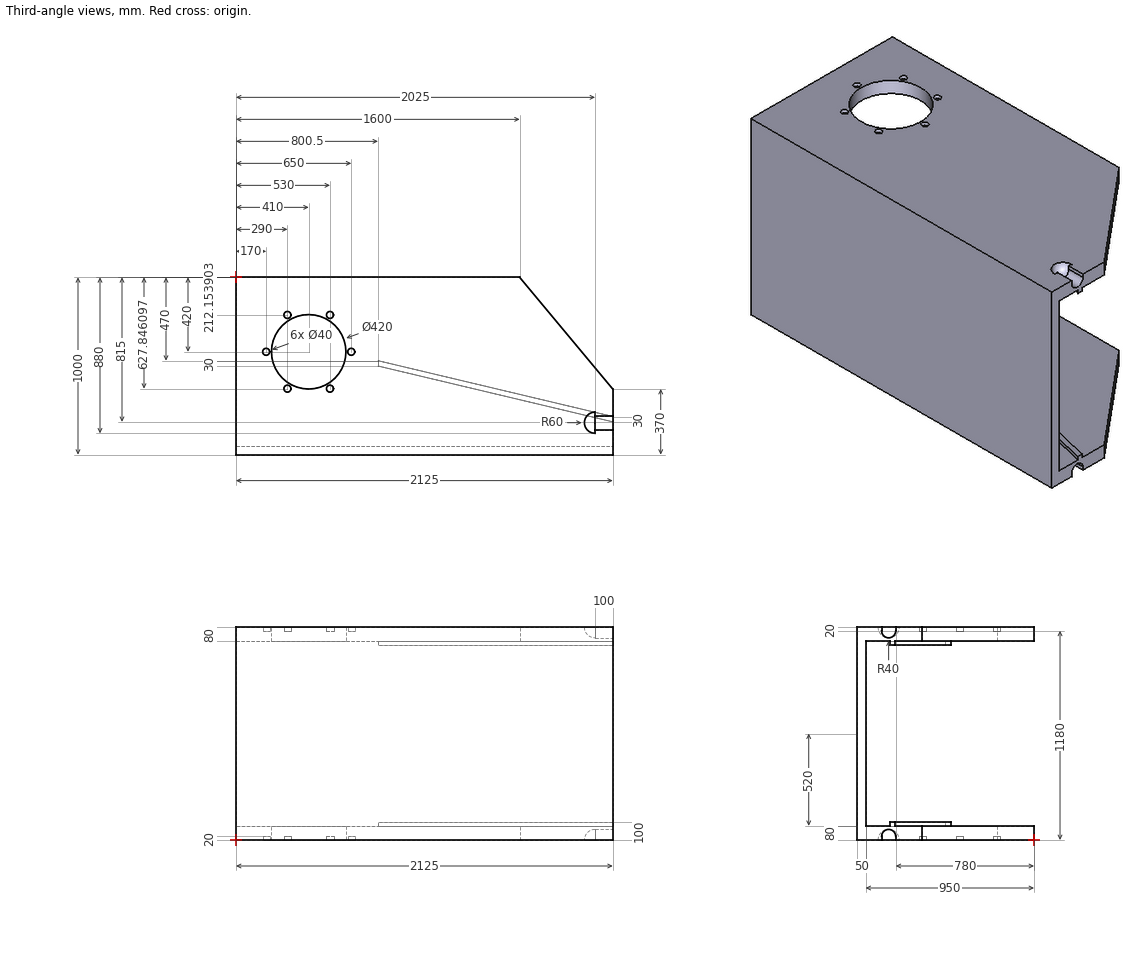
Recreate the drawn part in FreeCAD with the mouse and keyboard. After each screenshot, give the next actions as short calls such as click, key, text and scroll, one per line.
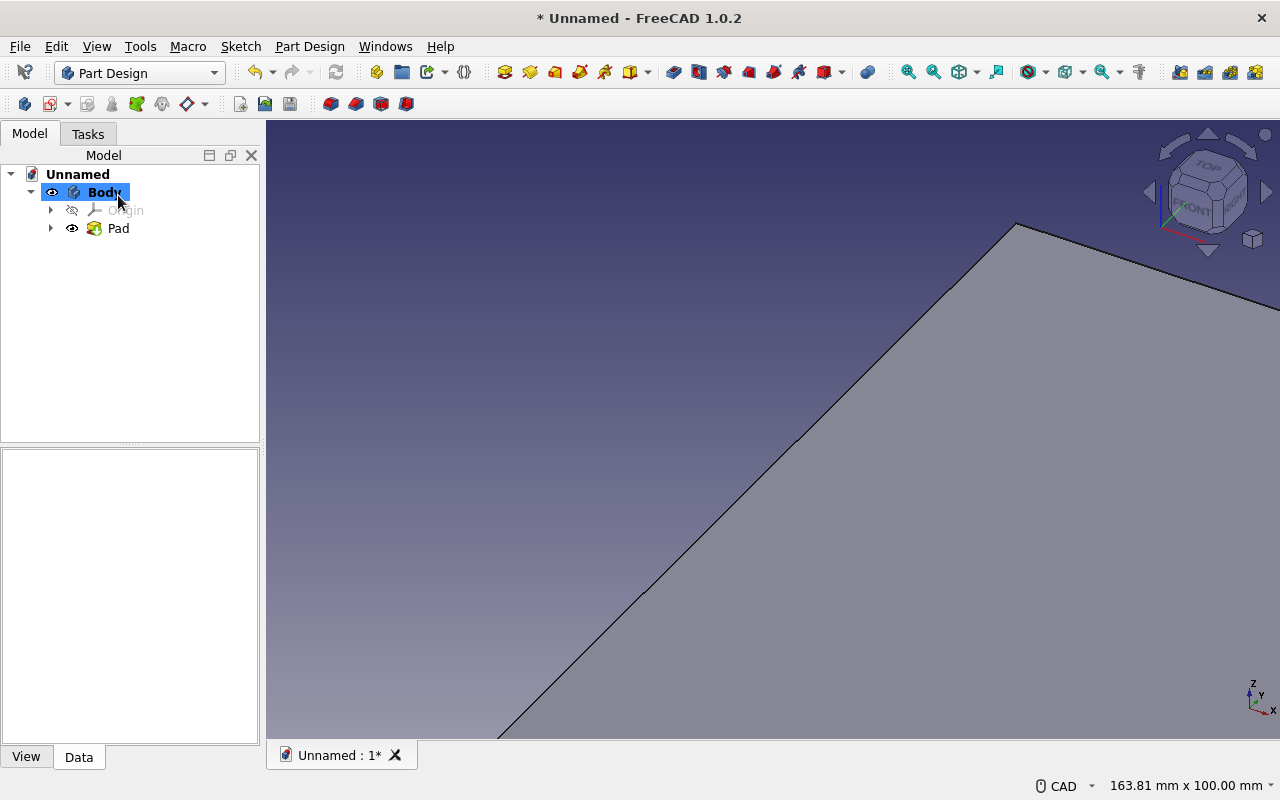
click(909, 72)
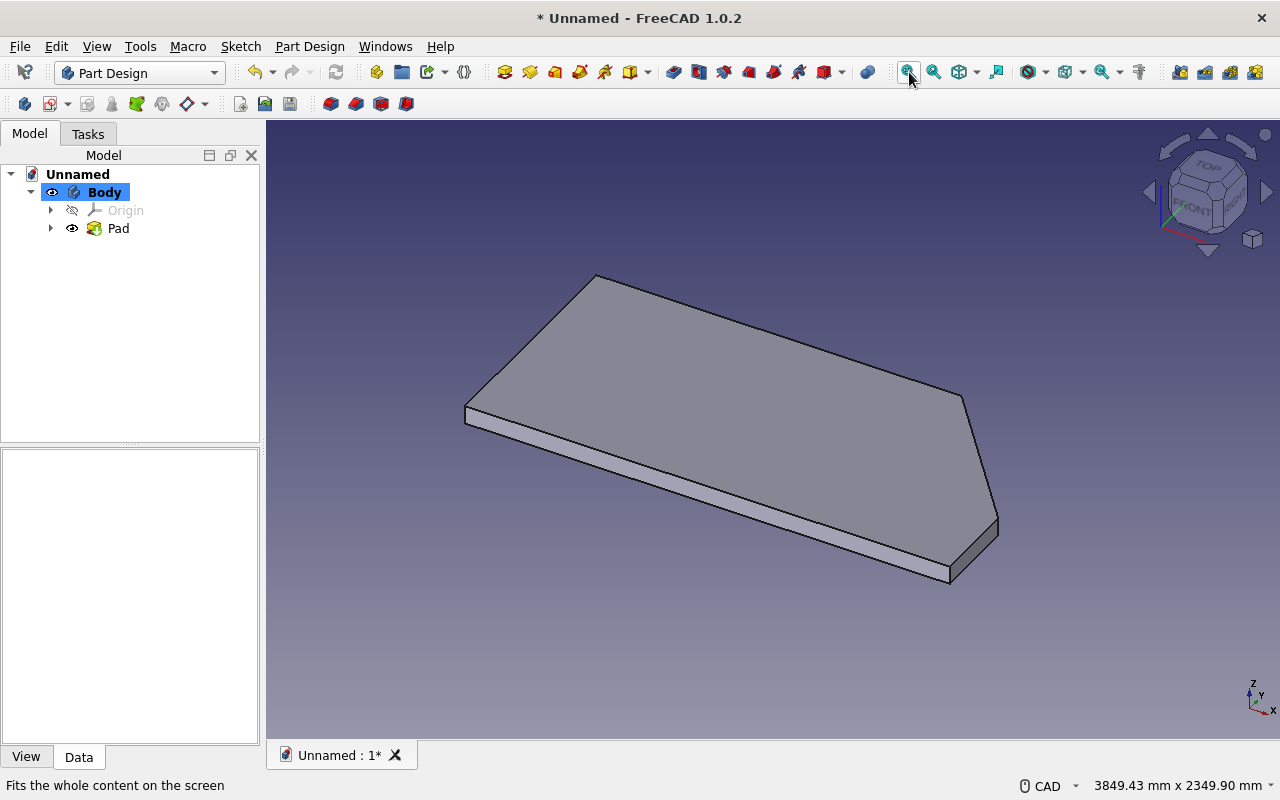
click(50, 104)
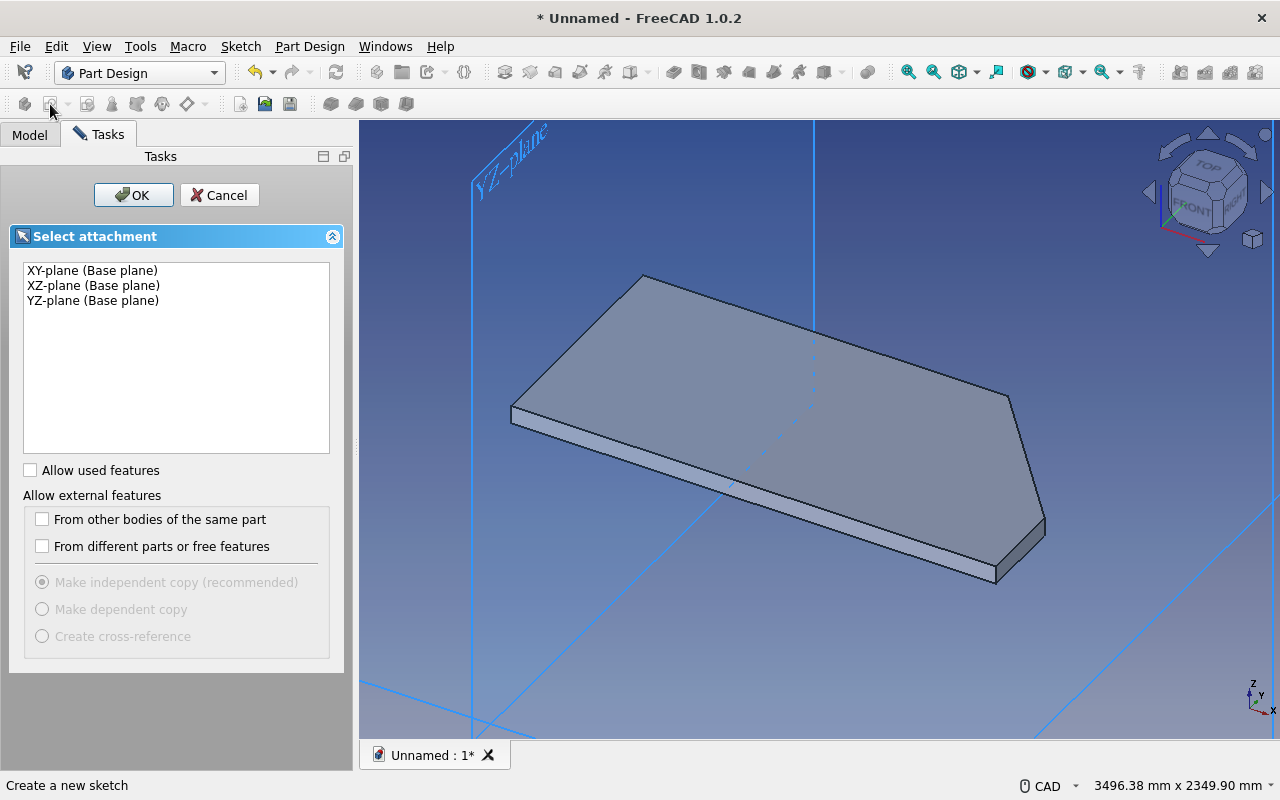
click(84, 300)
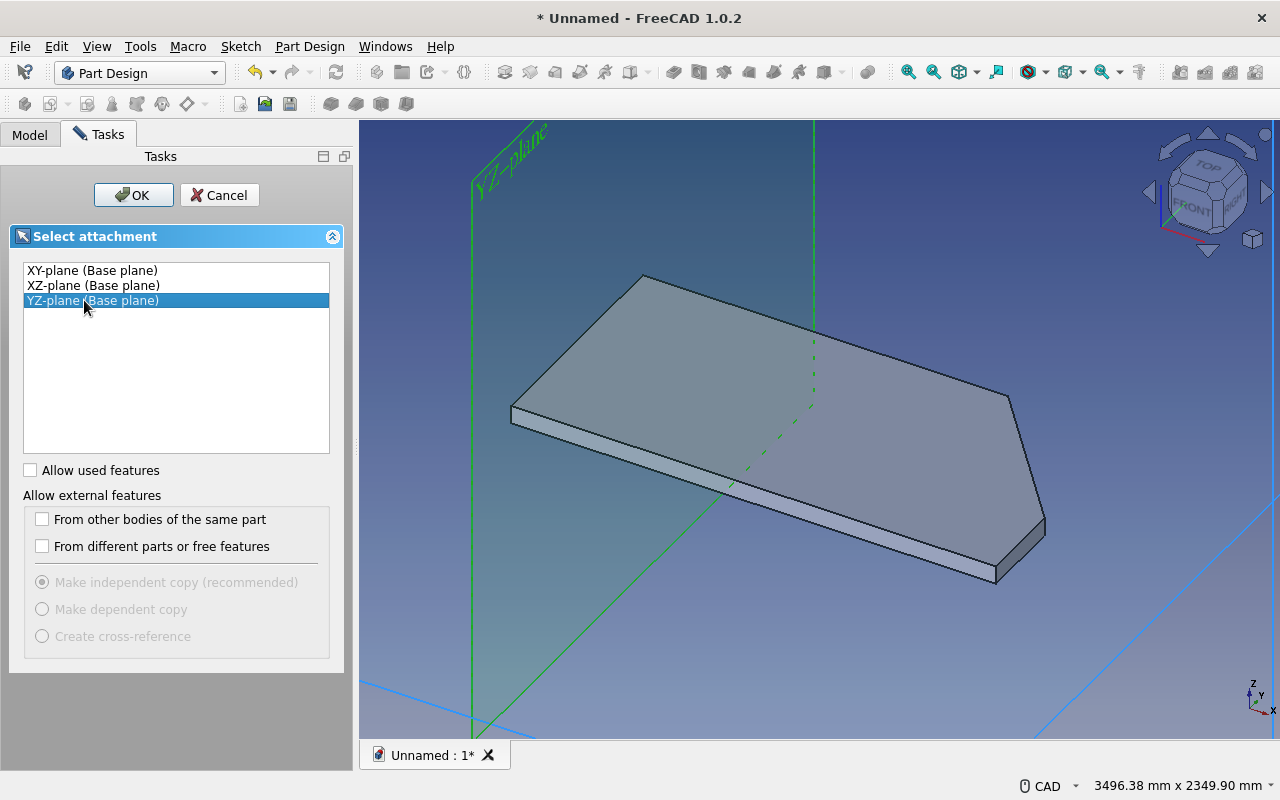
click(134, 195)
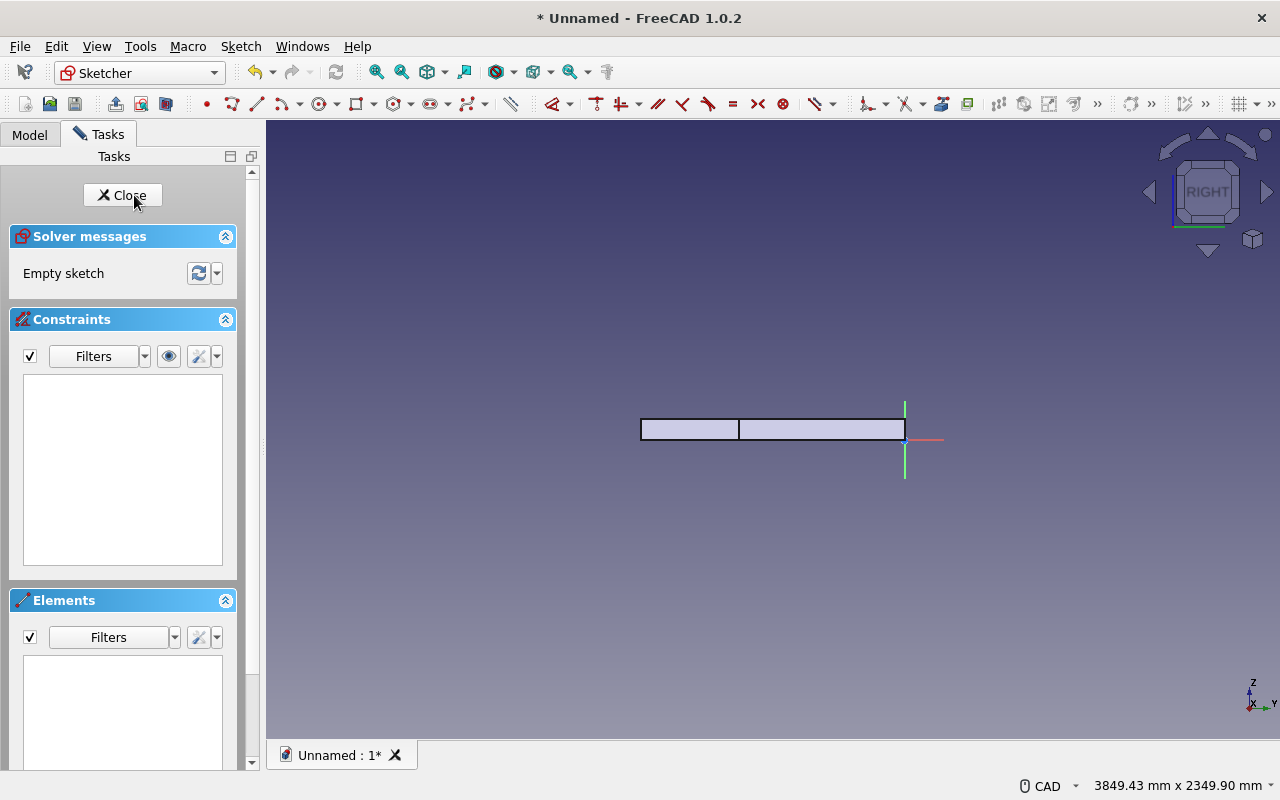
key(q)
key(s)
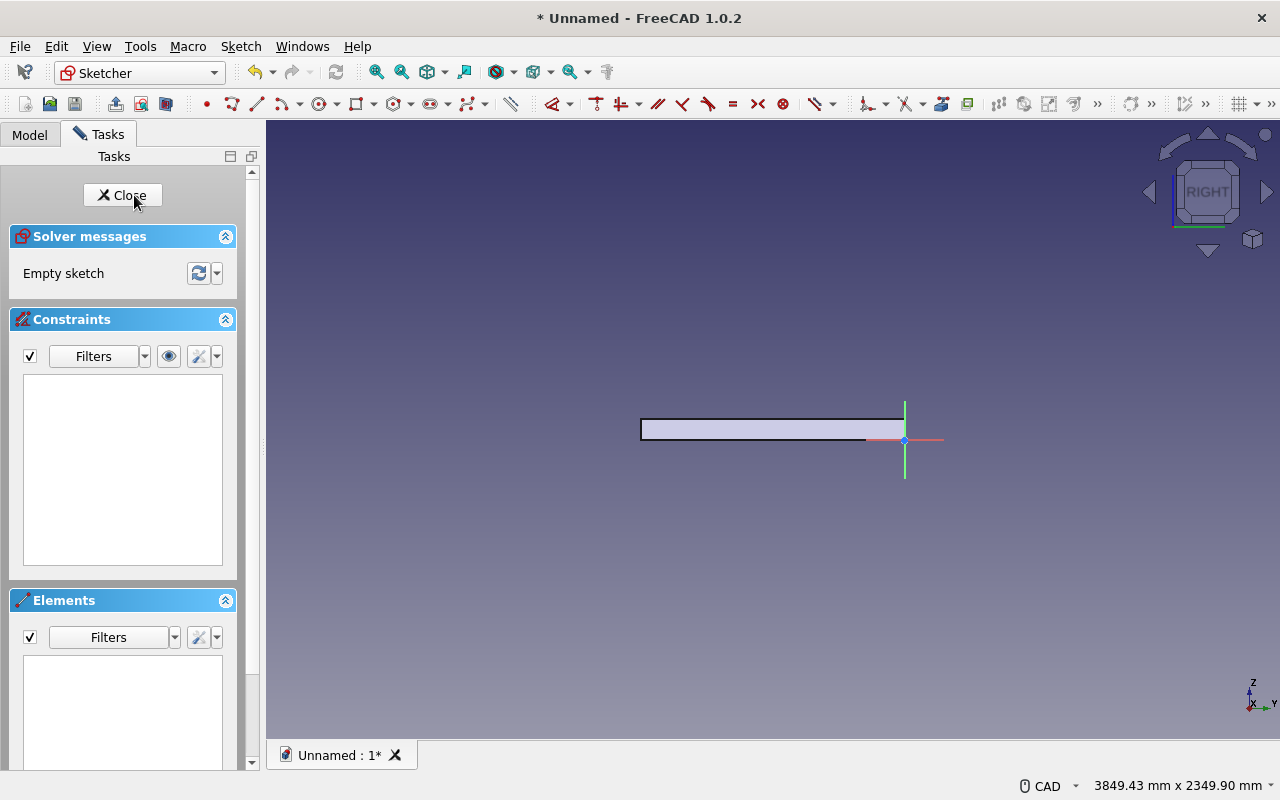
scroll(829, 305, up, 4)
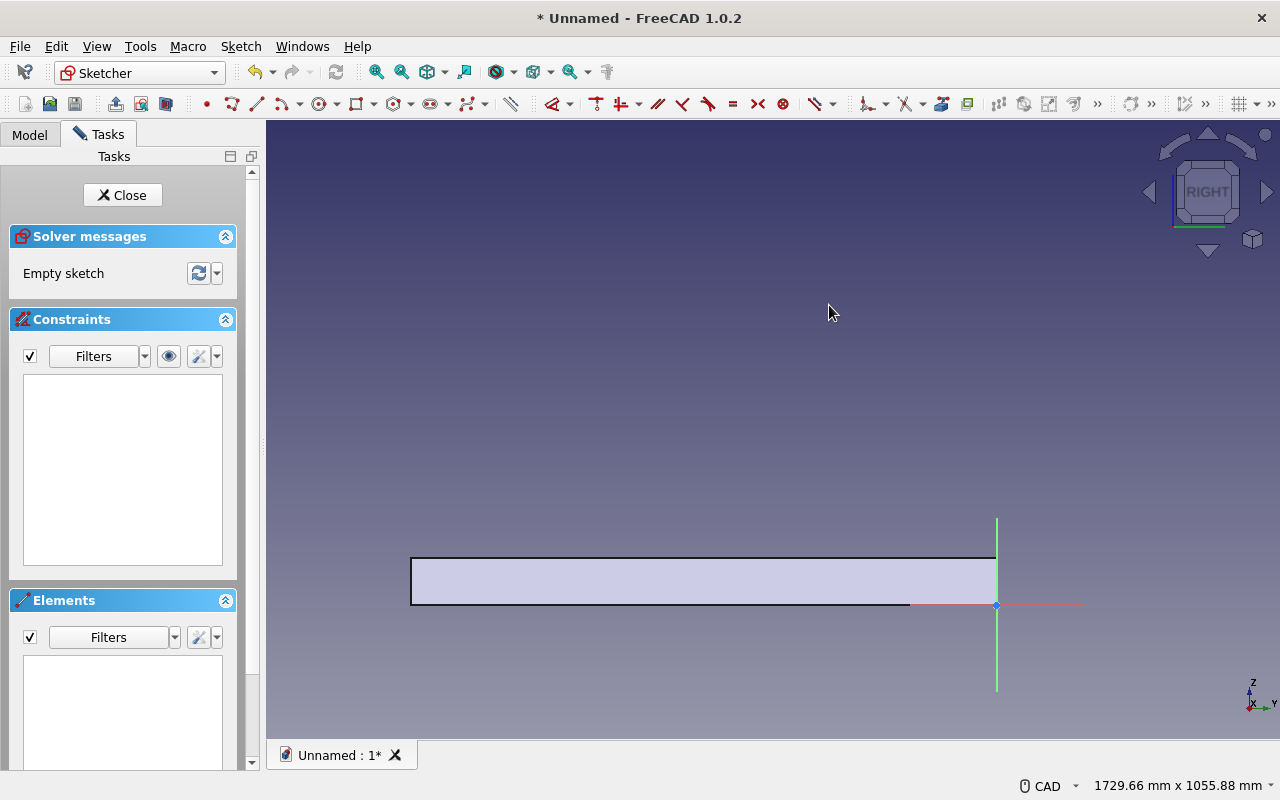
click(356, 104)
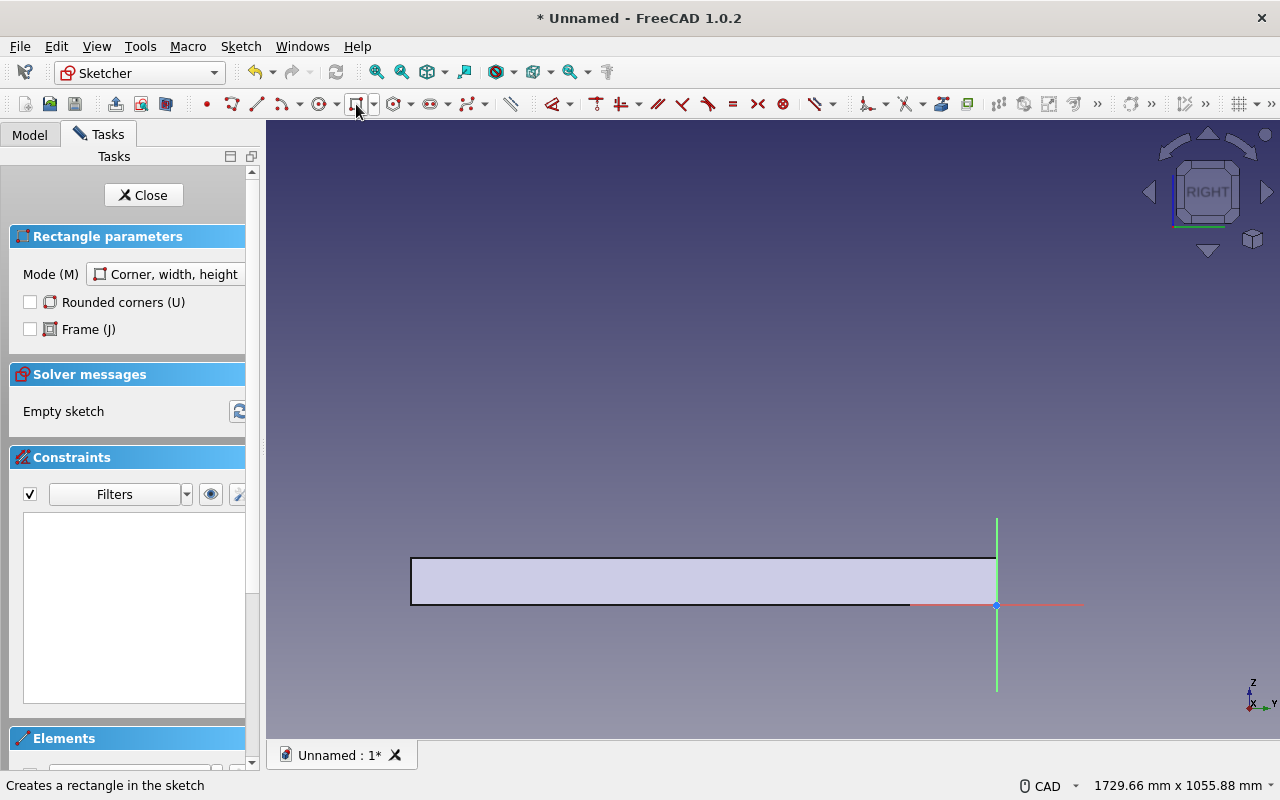
click(411, 253)
click(440, 558)
key(Escape)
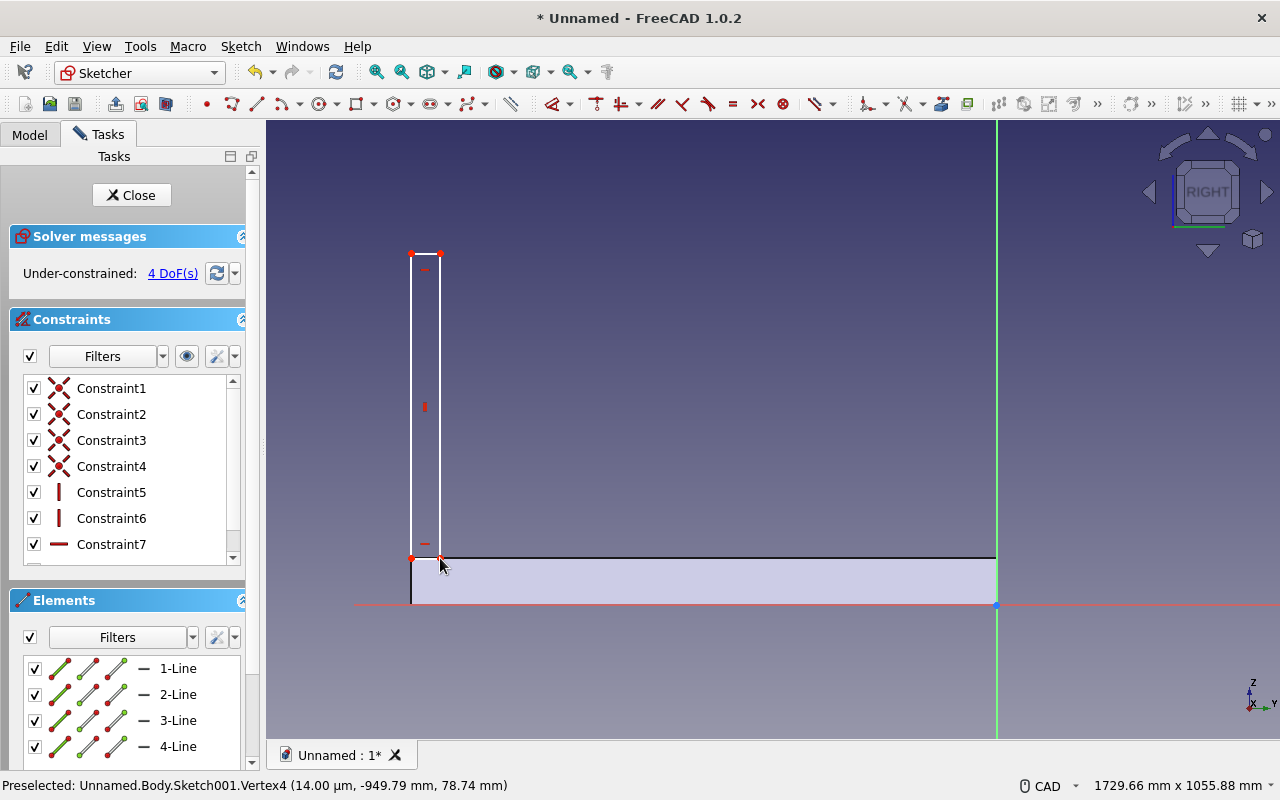
key(d)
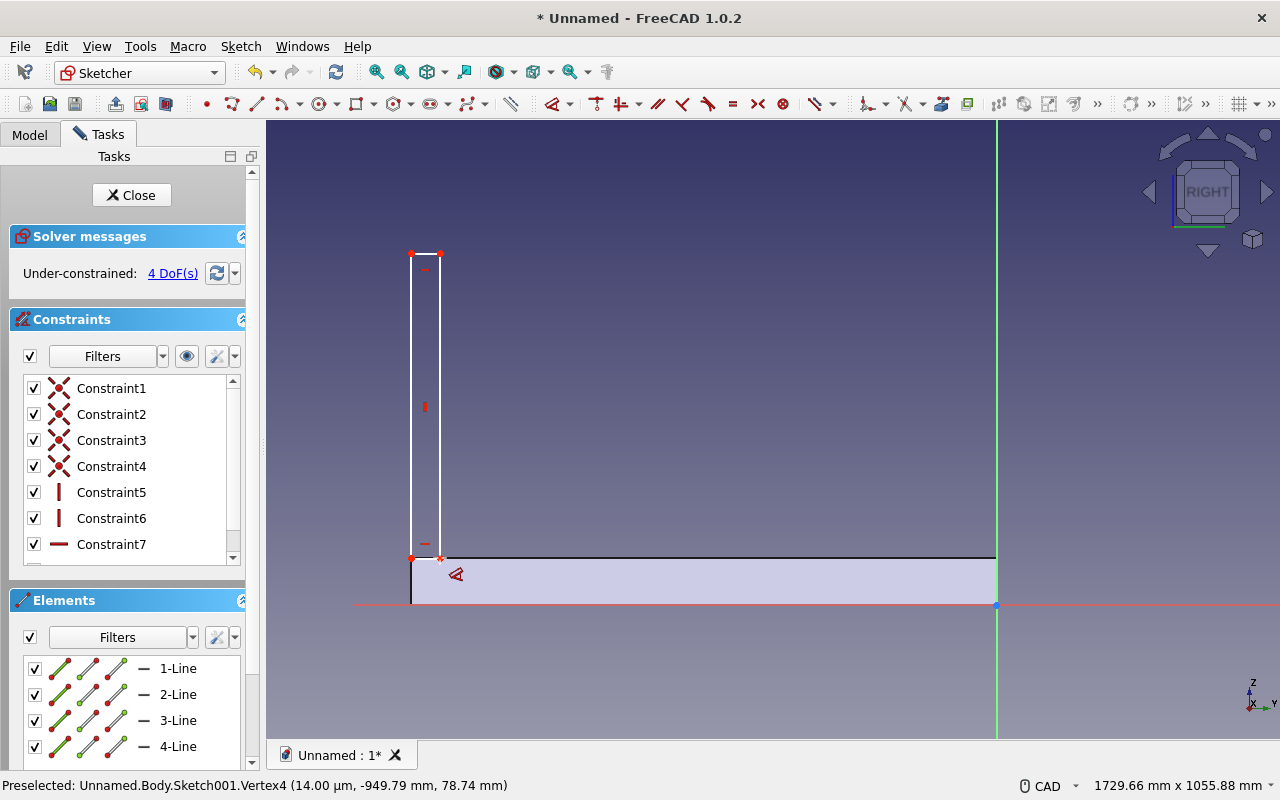
scroll(423, 559, up, 2)